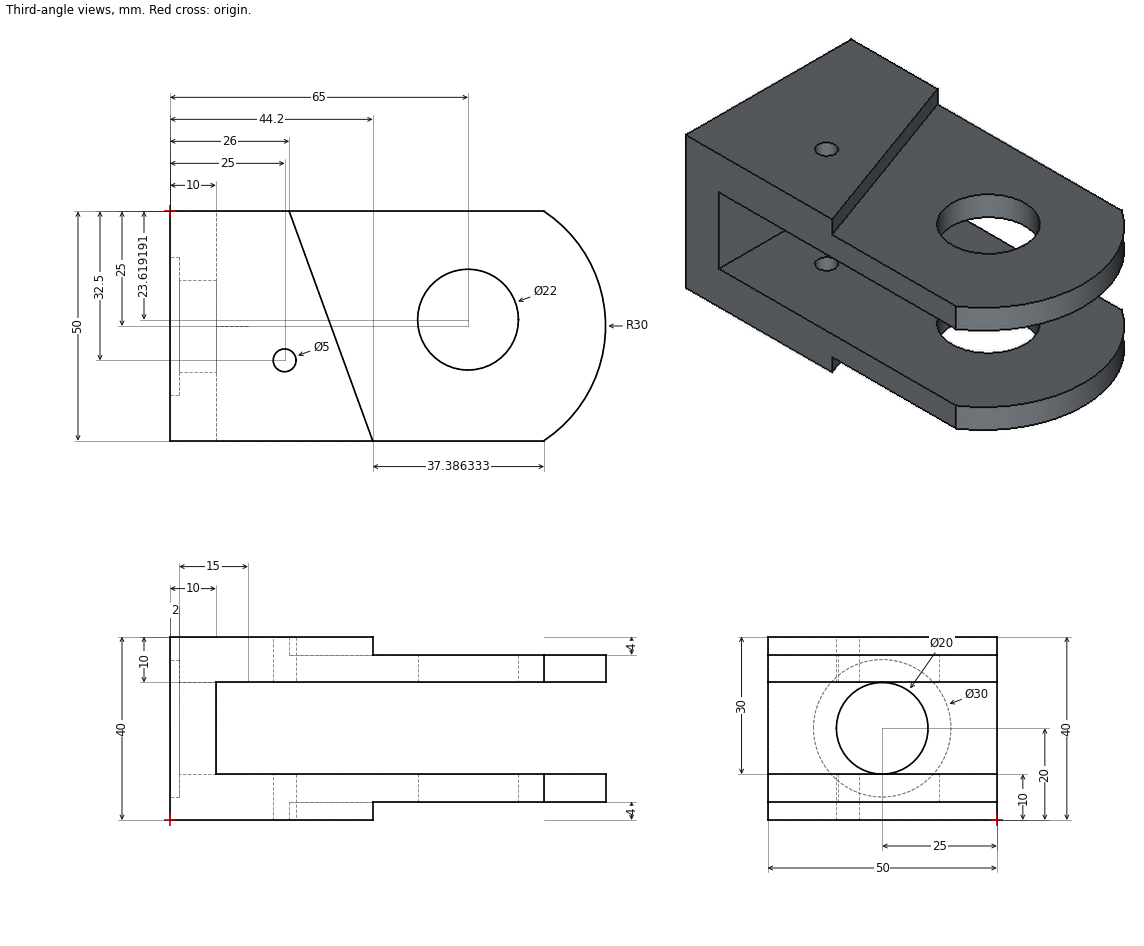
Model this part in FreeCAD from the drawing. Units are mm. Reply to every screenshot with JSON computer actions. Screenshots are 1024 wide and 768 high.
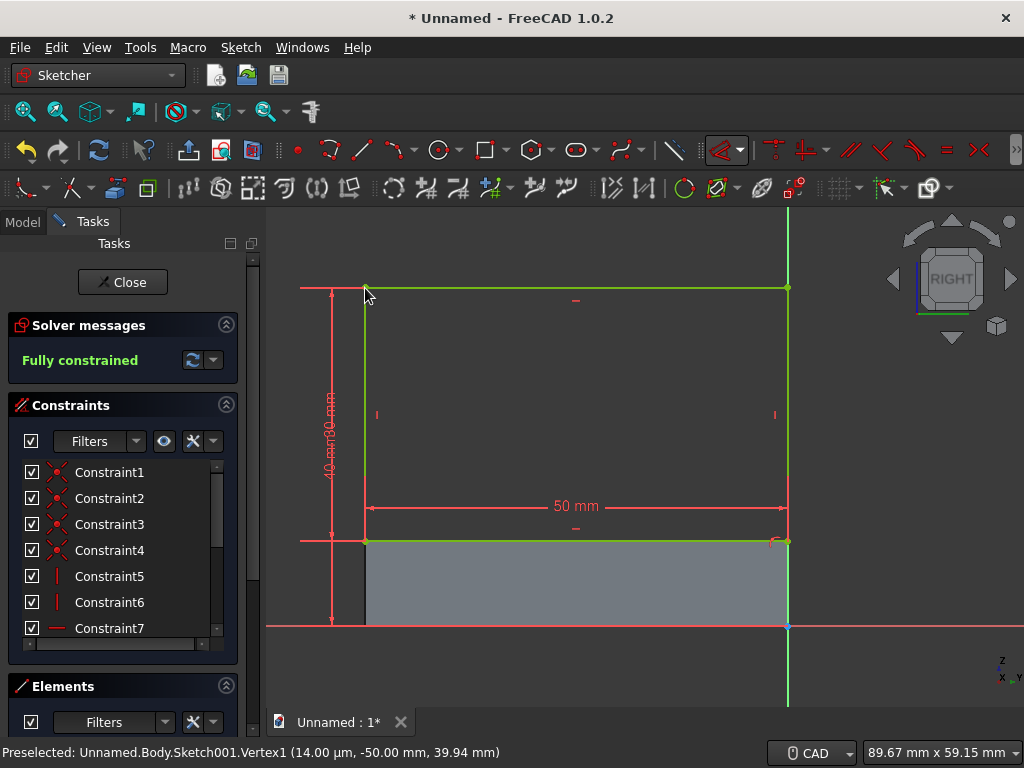
{"action": "left_click", "coordinate": [123, 282]}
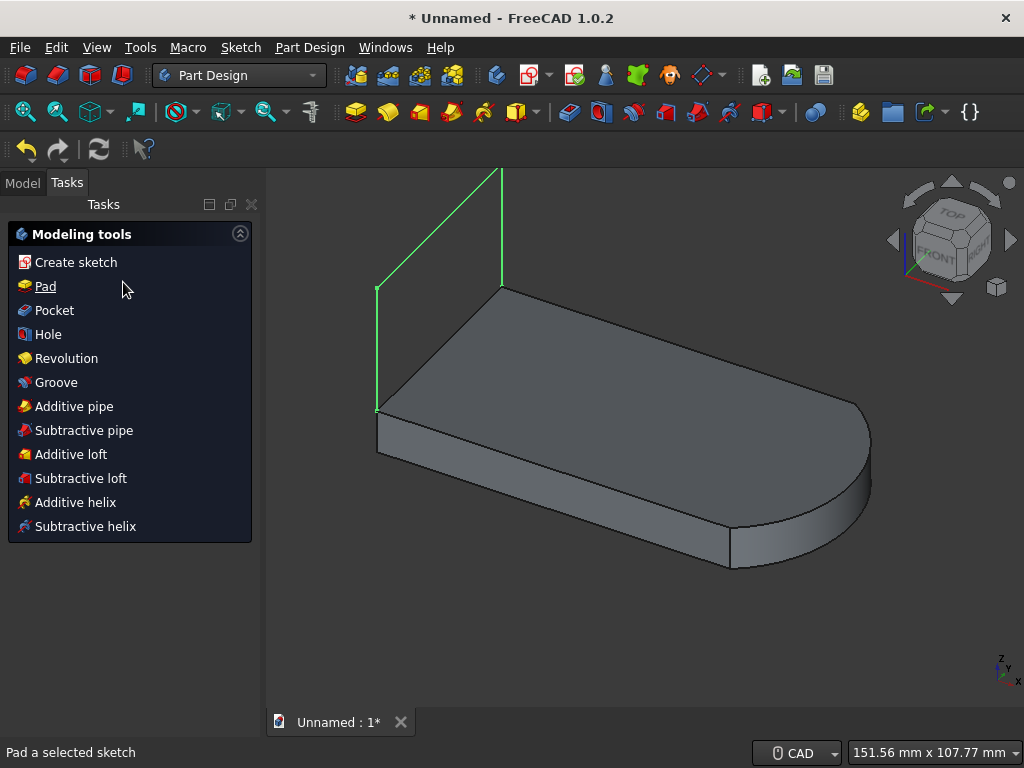
{"action": "left_click", "coordinate": [356, 112]}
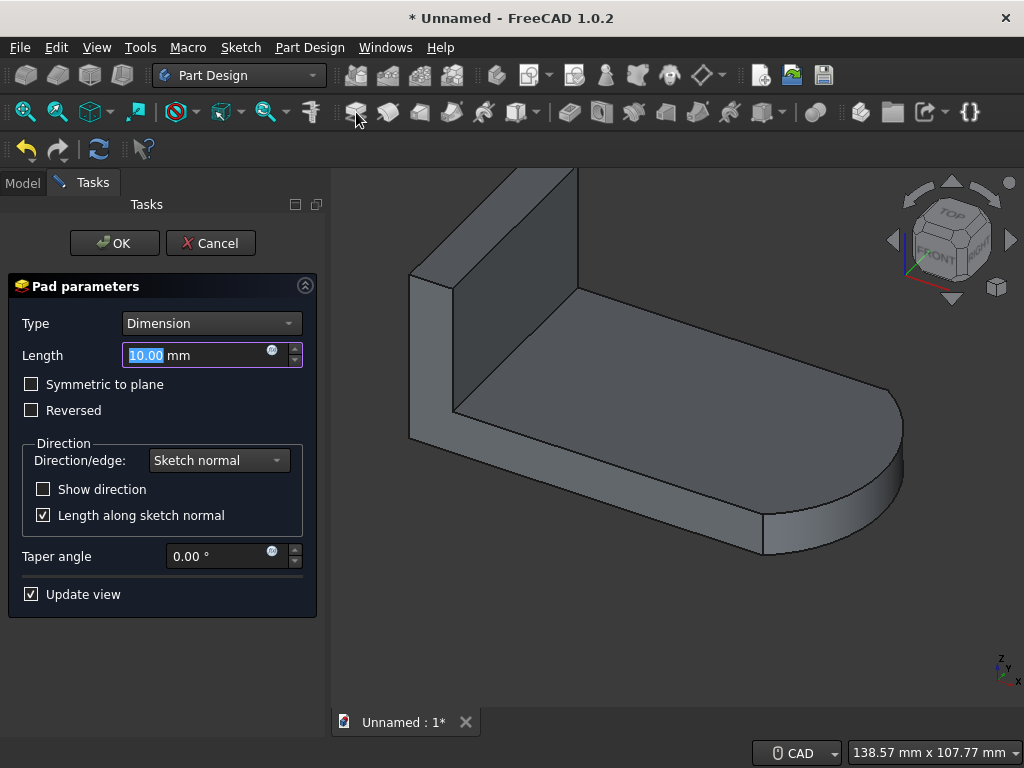
{"action": "type", "text": "10"}
{"action": "key", "text": "Tab"}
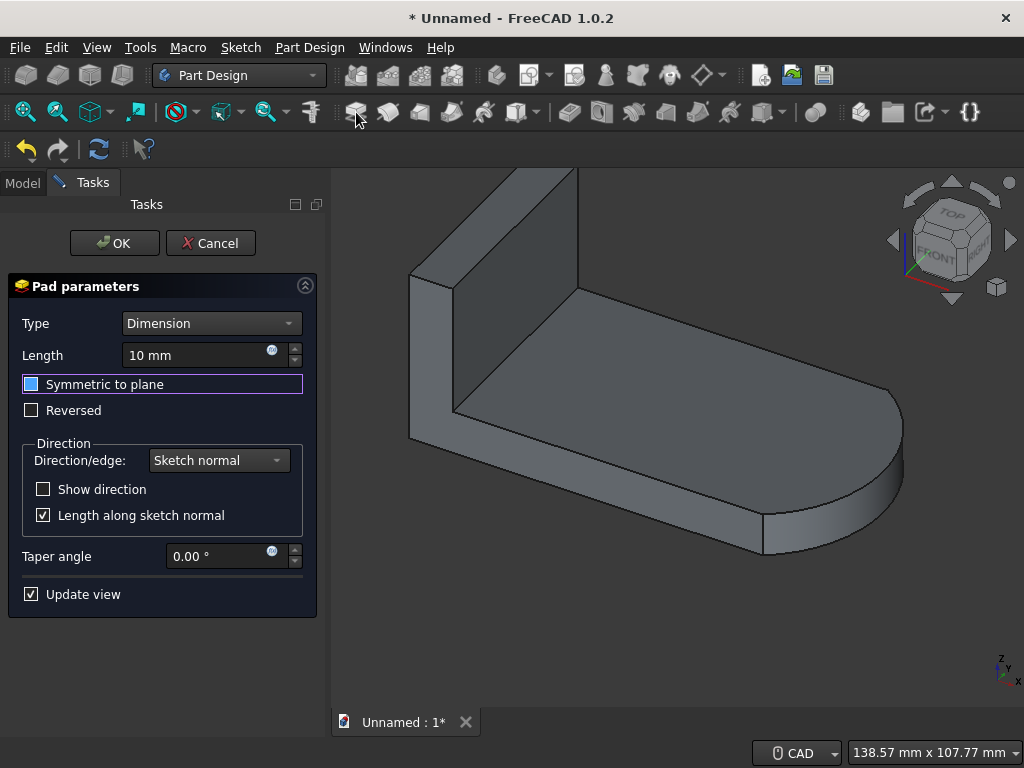
{"action": "left_click", "coordinate": [115, 243]}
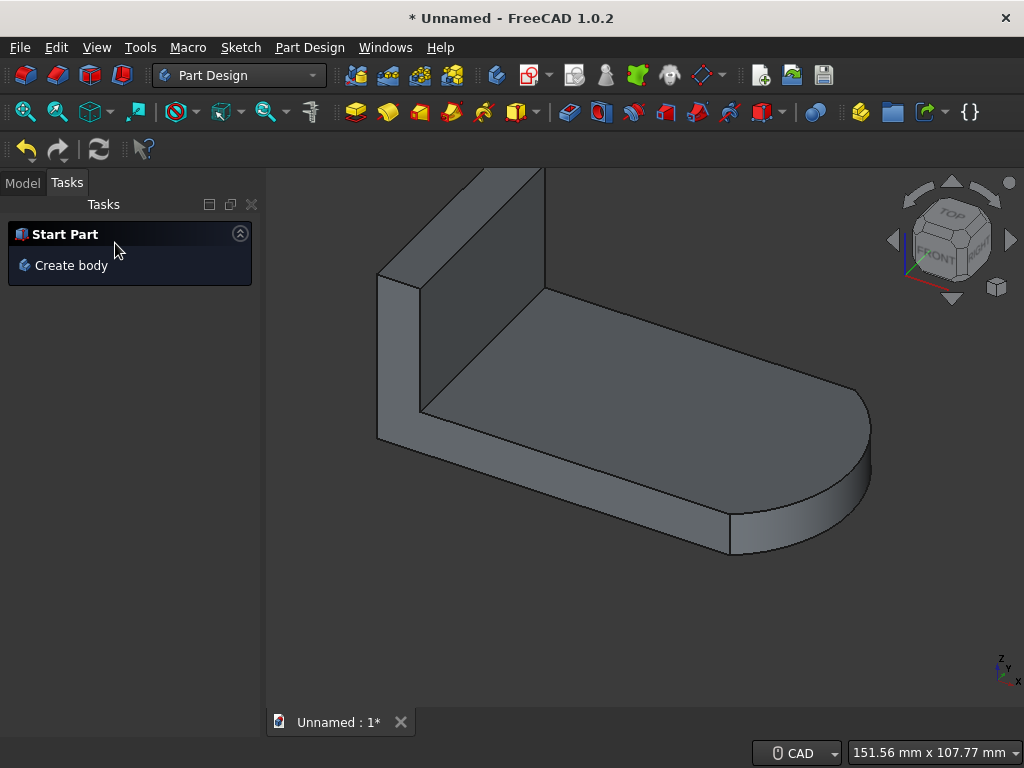
{"action": "key", "text": "v f"}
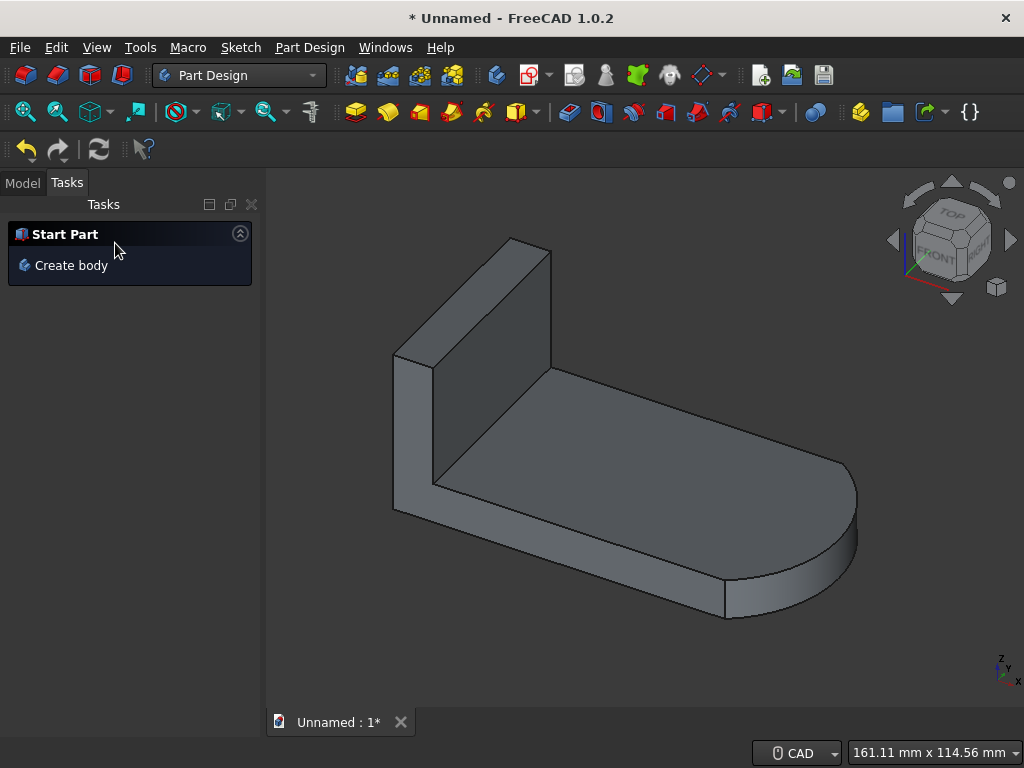
{"action": "left_click", "coordinate": [23, 182]}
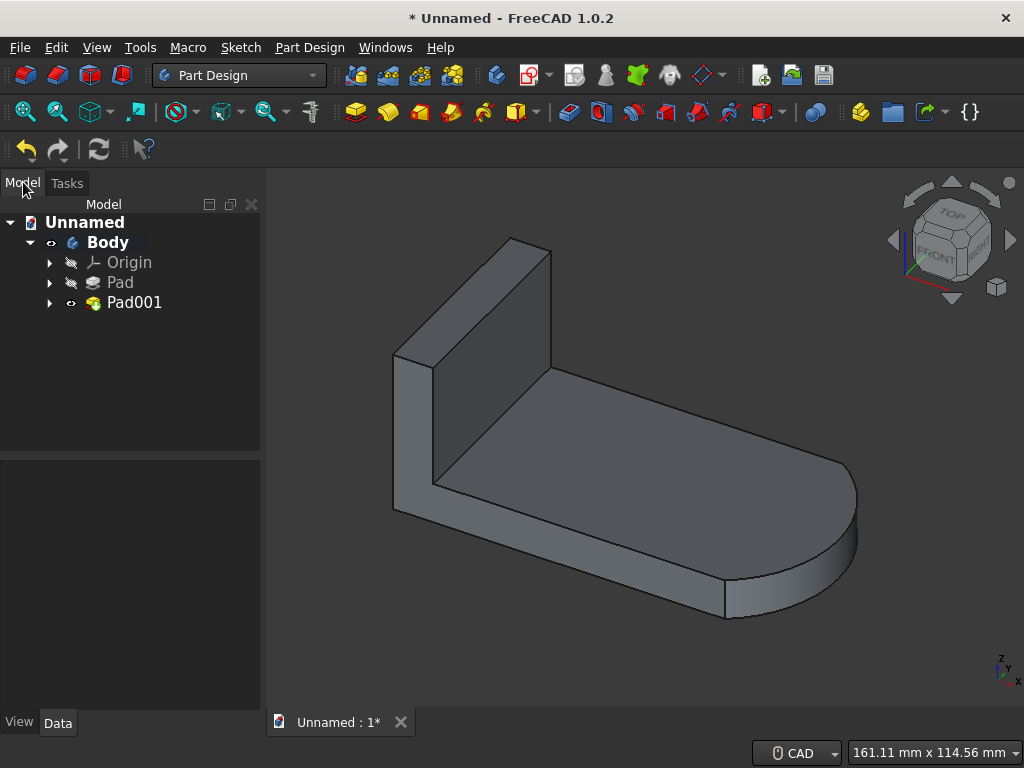
{"action": "left_click", "coordinate": [50, 263]}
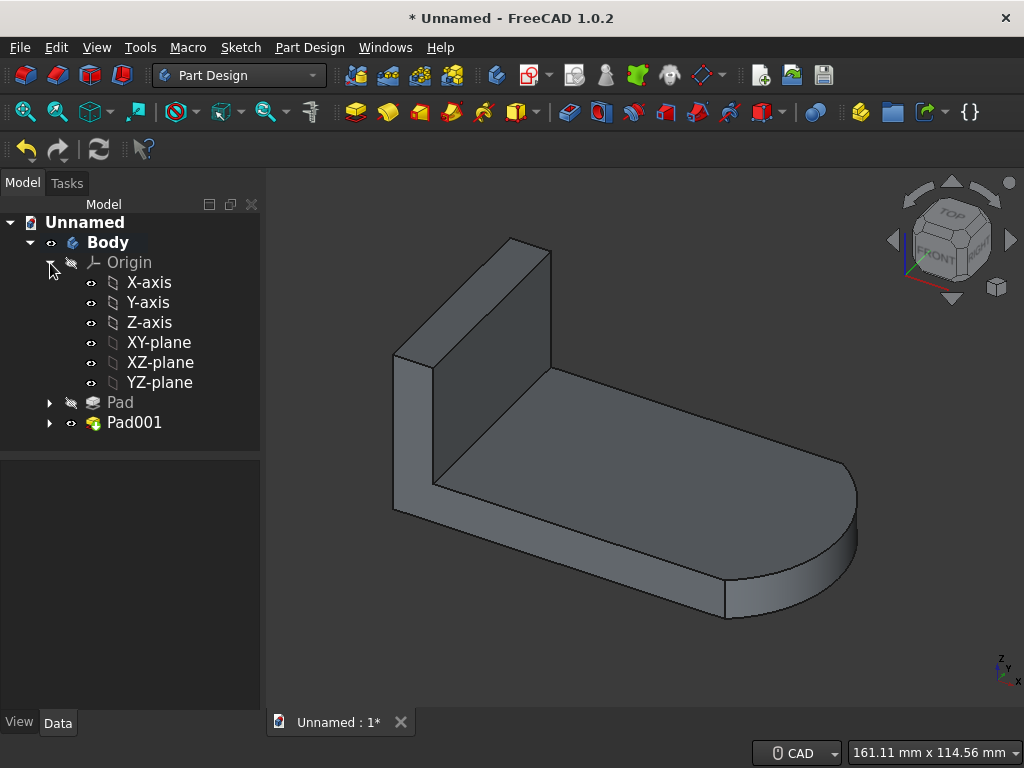
{"action": "left_click", "coordinate": [136, 343]}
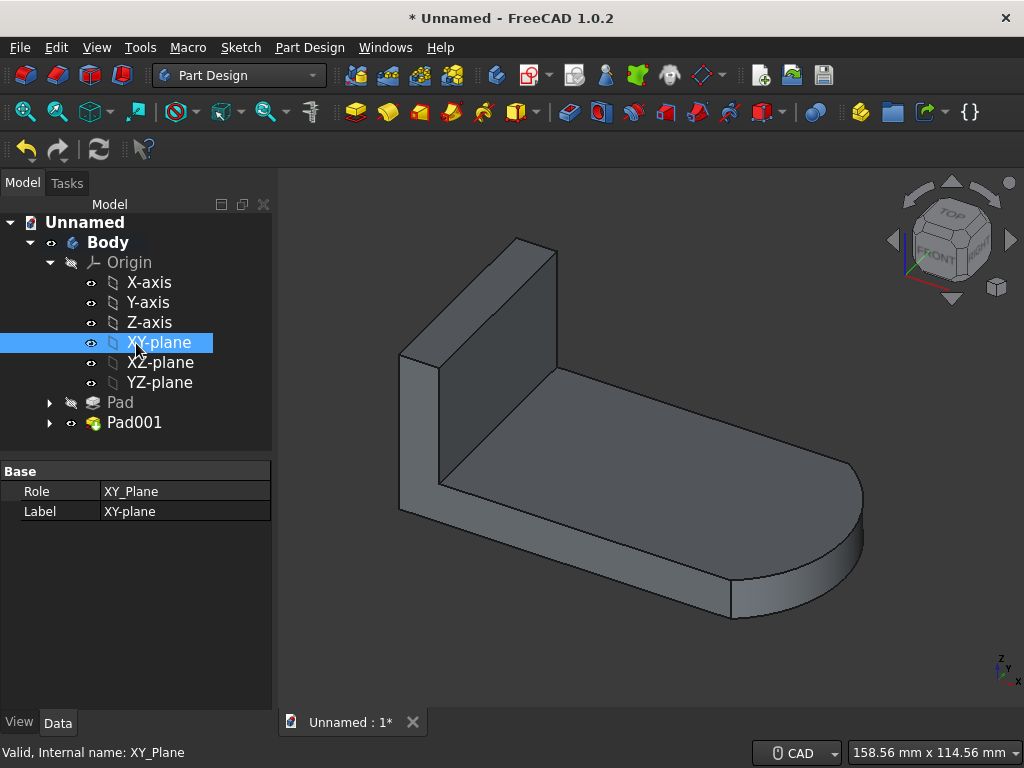
{"action": "left_click", "coordinate": [702, 76]}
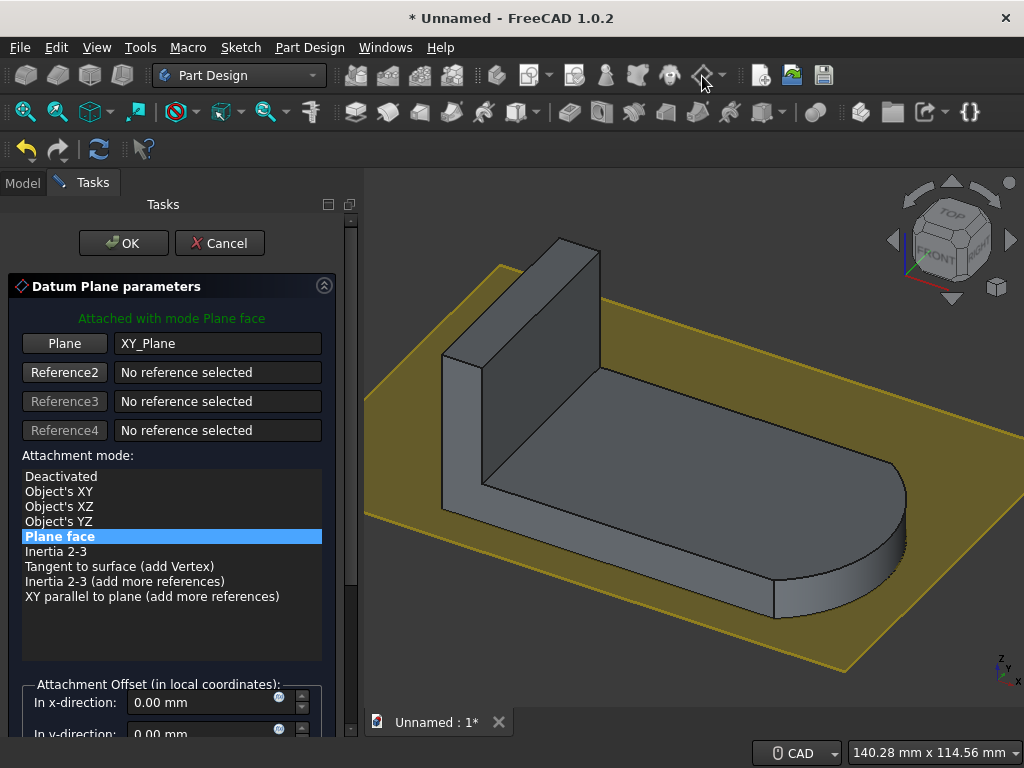
{"action": "scroll", "coordinate": [351, 475], "scroll_direction": "down", "scroll_amount": 2}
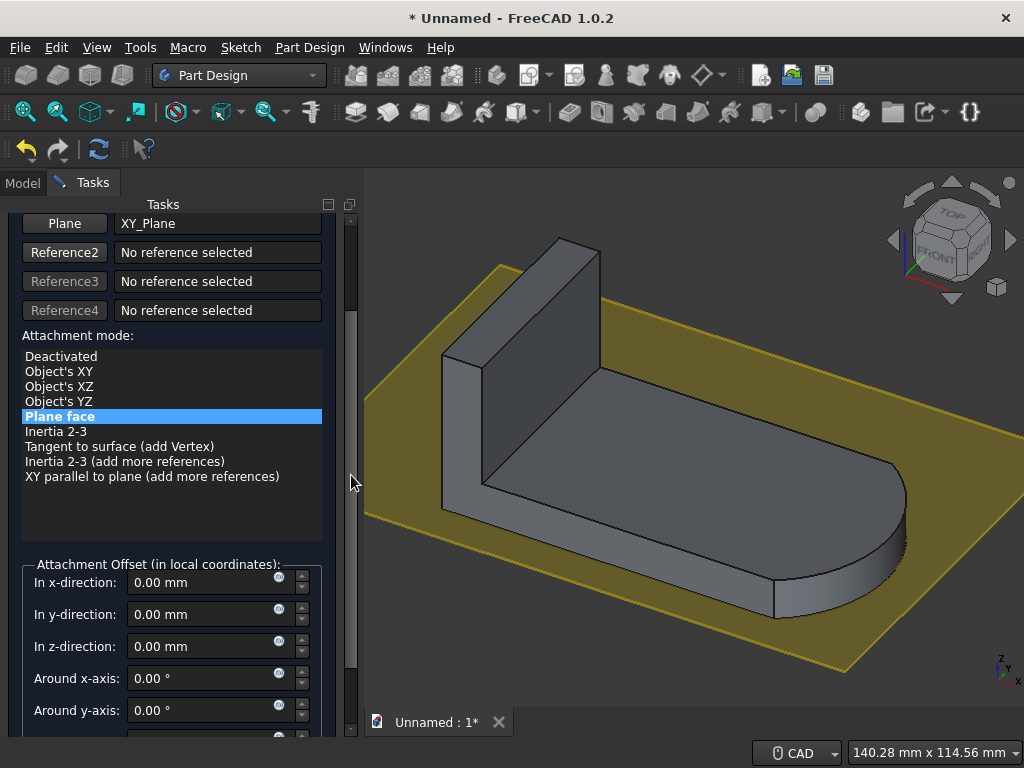
{"action": "triple_click", "coordinate": [210, 646]}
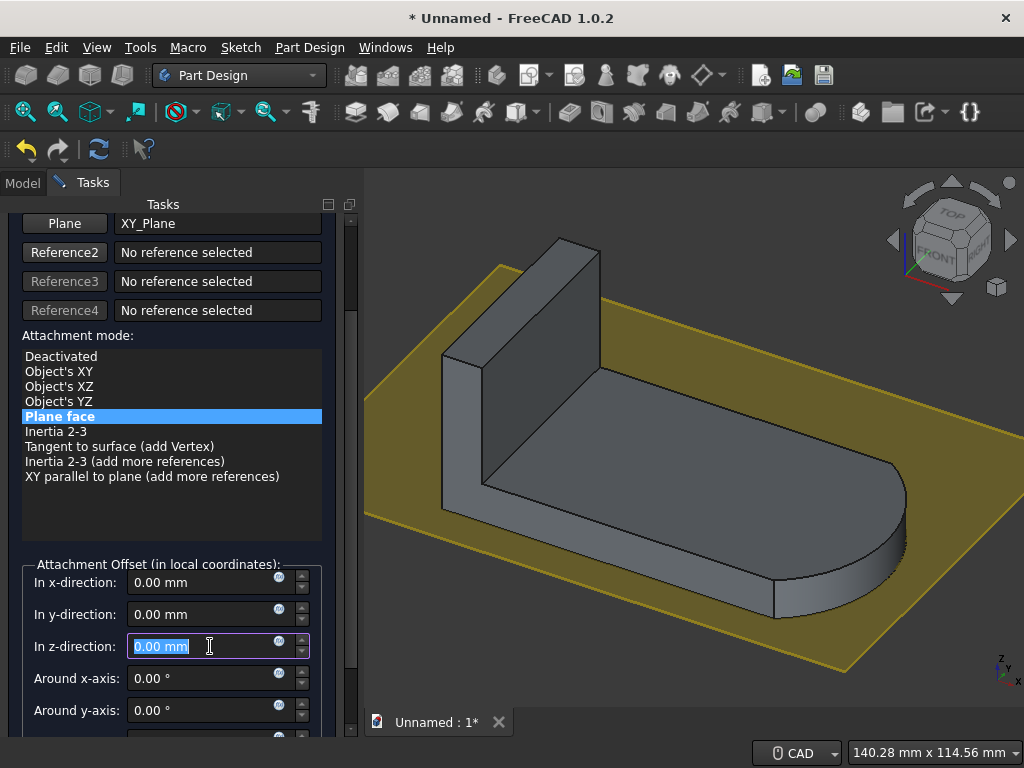
{"action": "type", "text": "30"}
{"action": "key", "text": "Tab"}